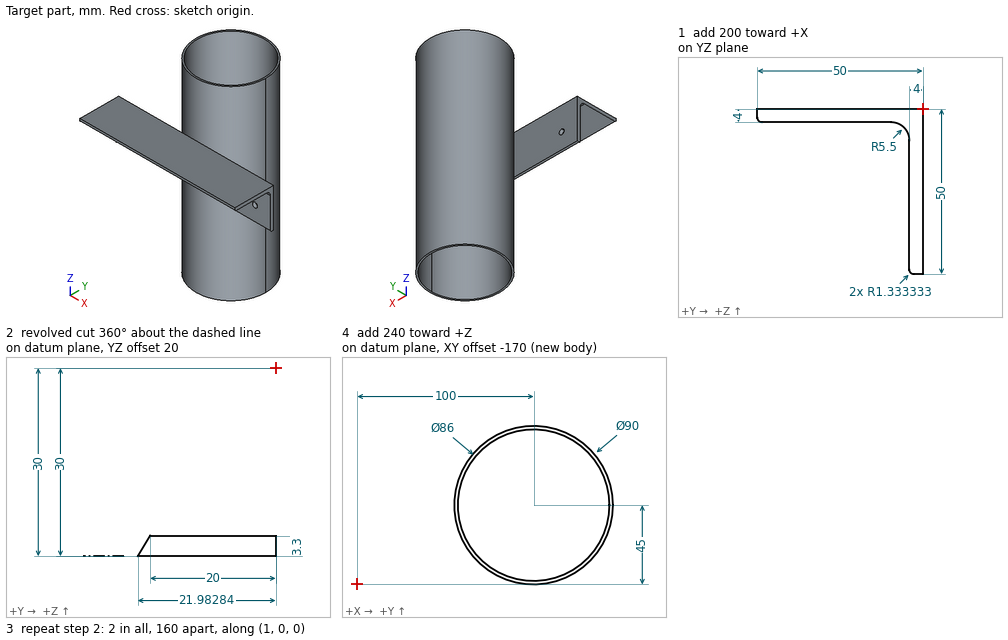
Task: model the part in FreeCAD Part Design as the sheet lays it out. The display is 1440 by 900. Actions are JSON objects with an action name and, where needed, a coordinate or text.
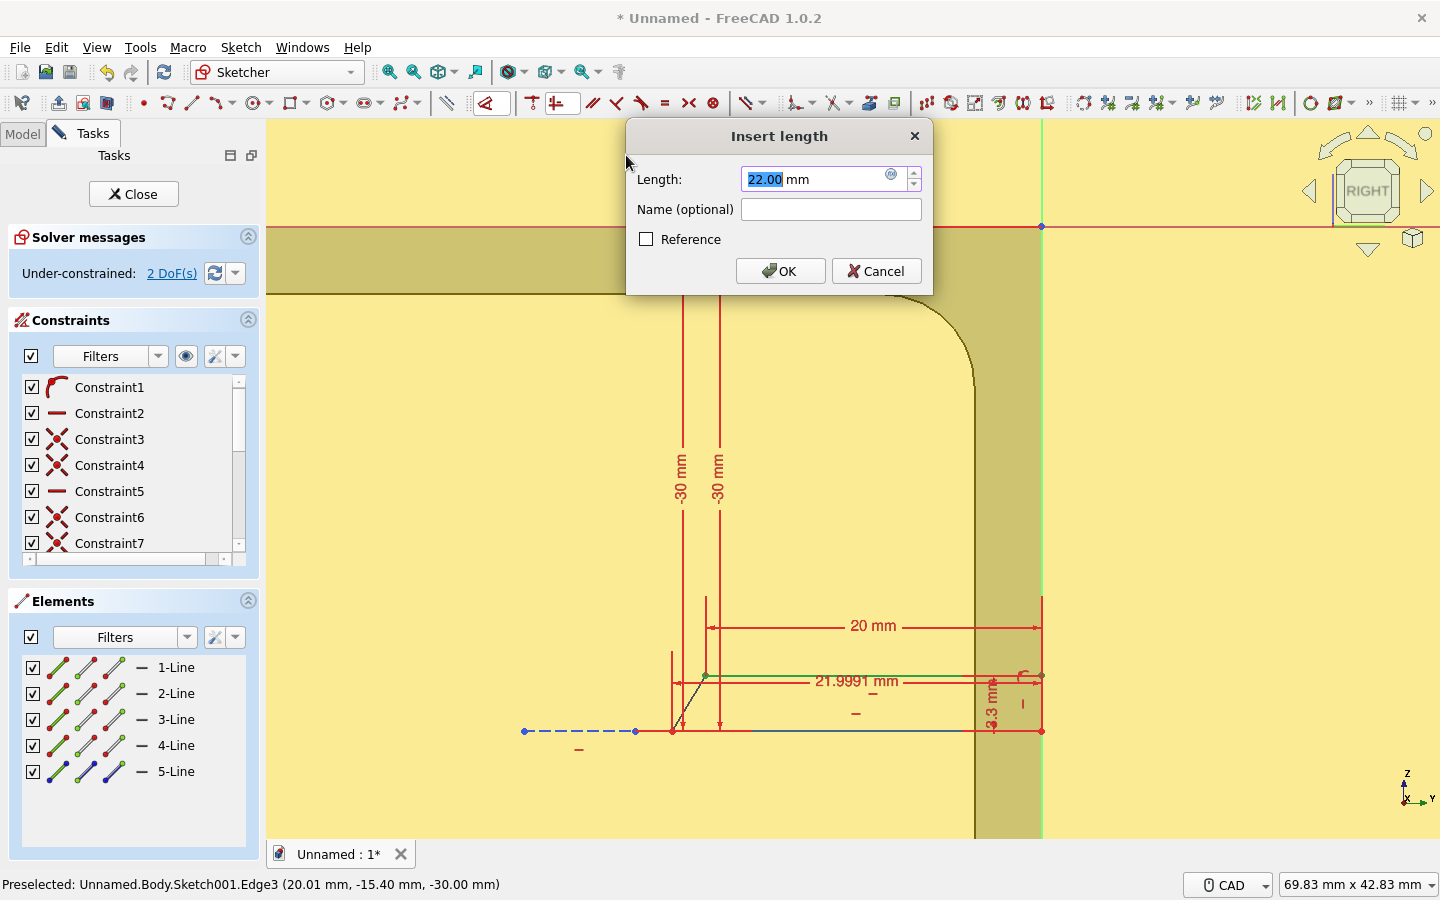
{"action": "type", "text": "21.98284"}
{"action": "key", "text": "Return"}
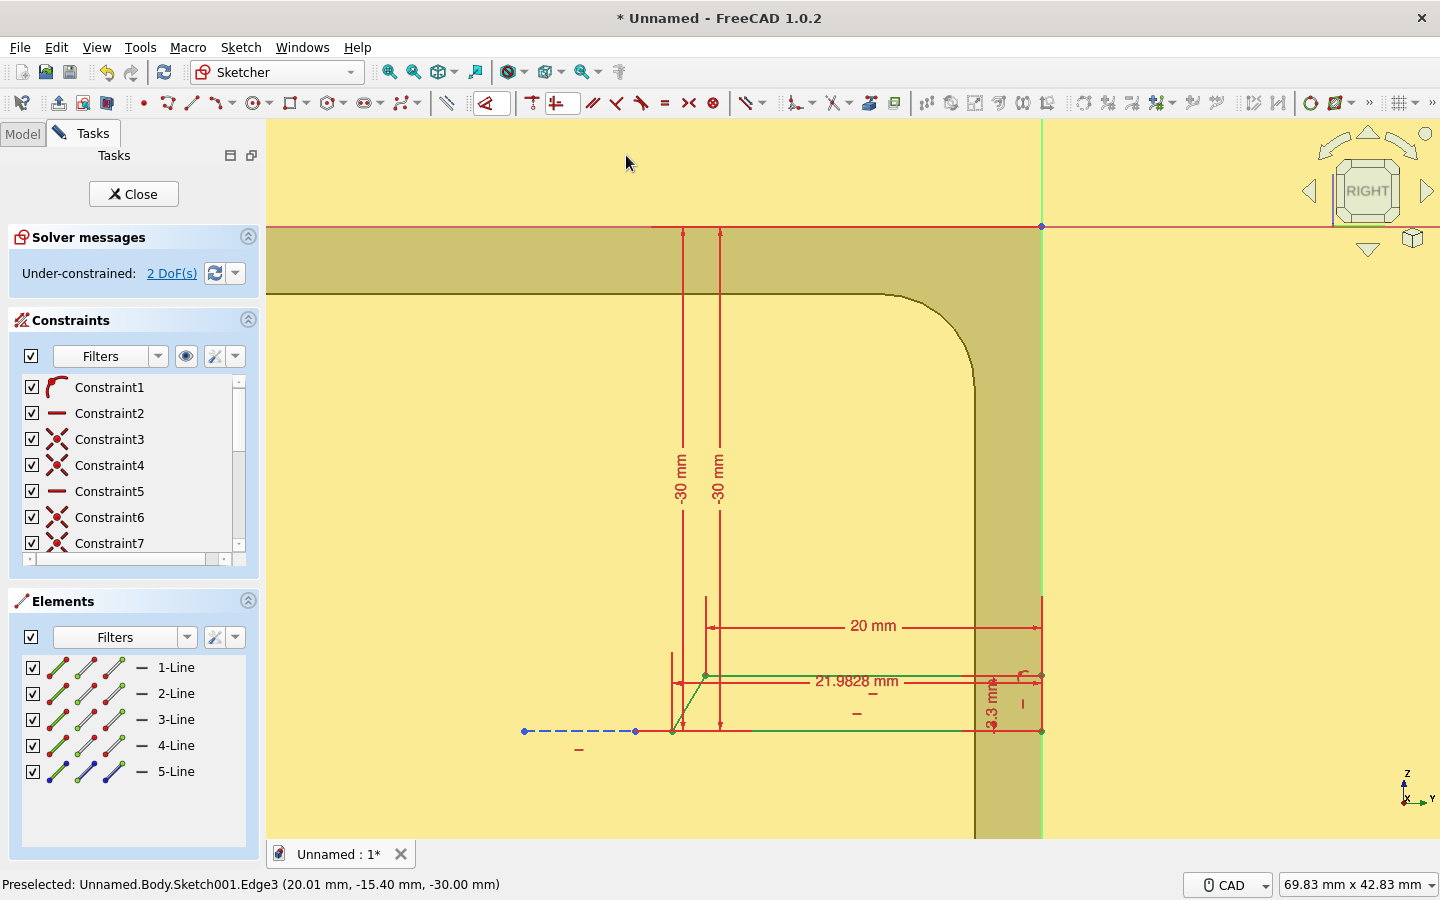
{"action": "left_click", "coordinate": [134, 194]}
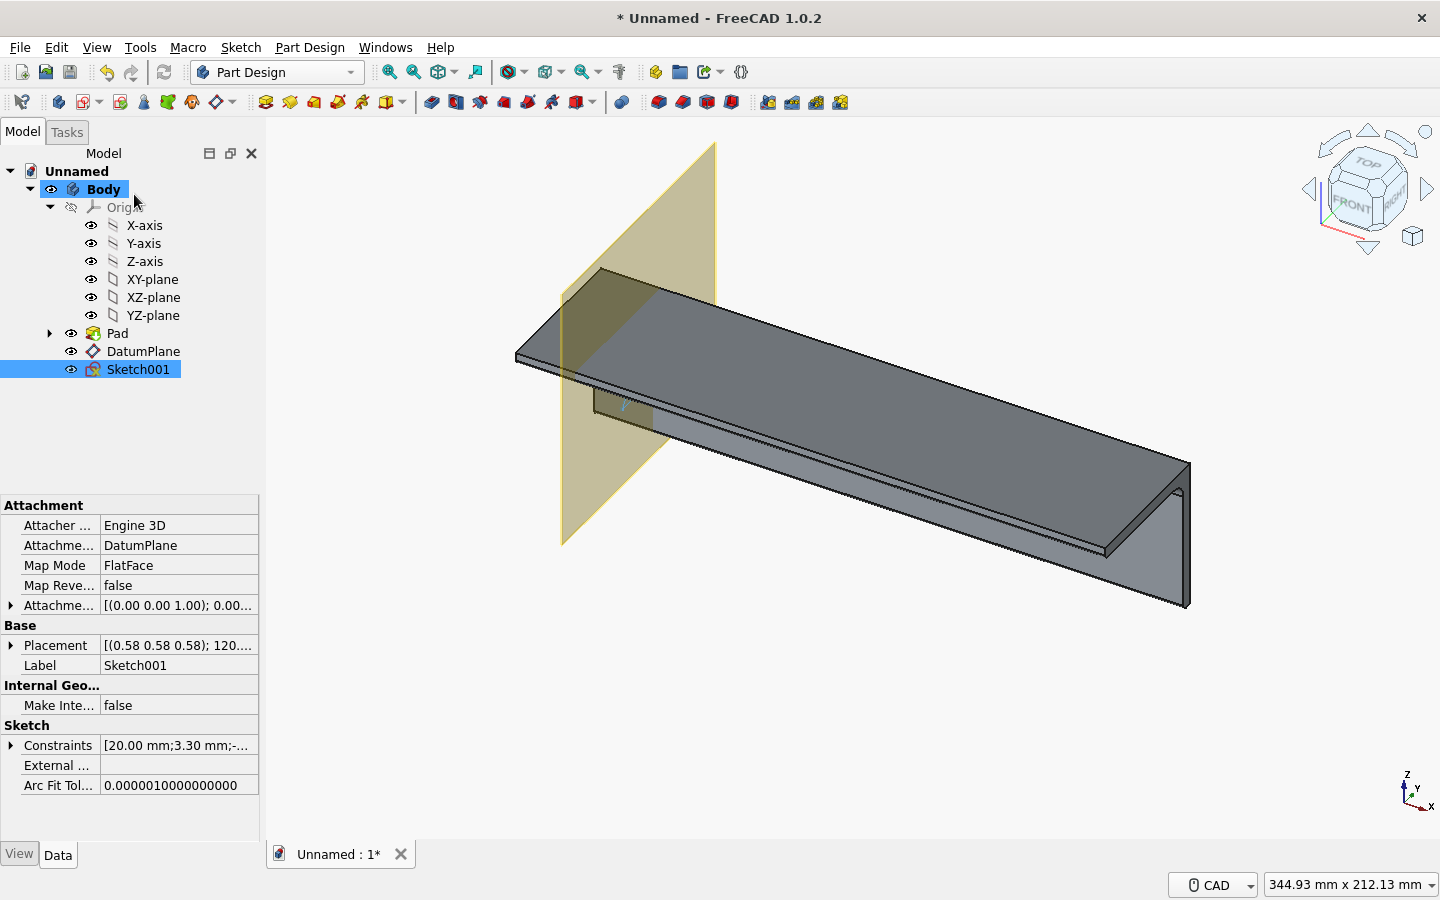
{"action": "left_click", "coordinate": [480, 102]}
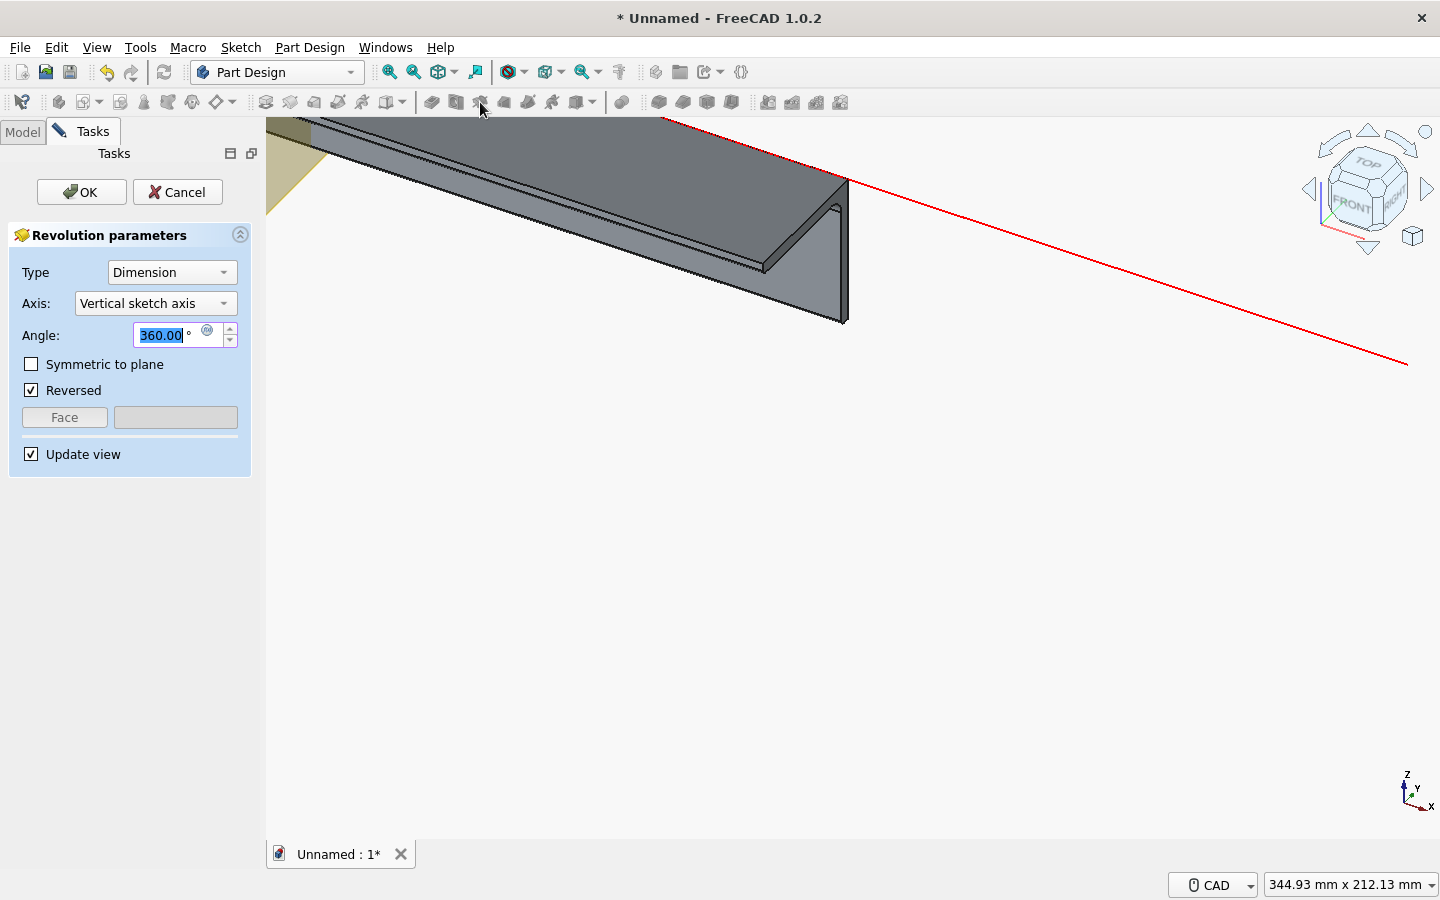
{"action": "left_click", "coordinate": [156, 304]}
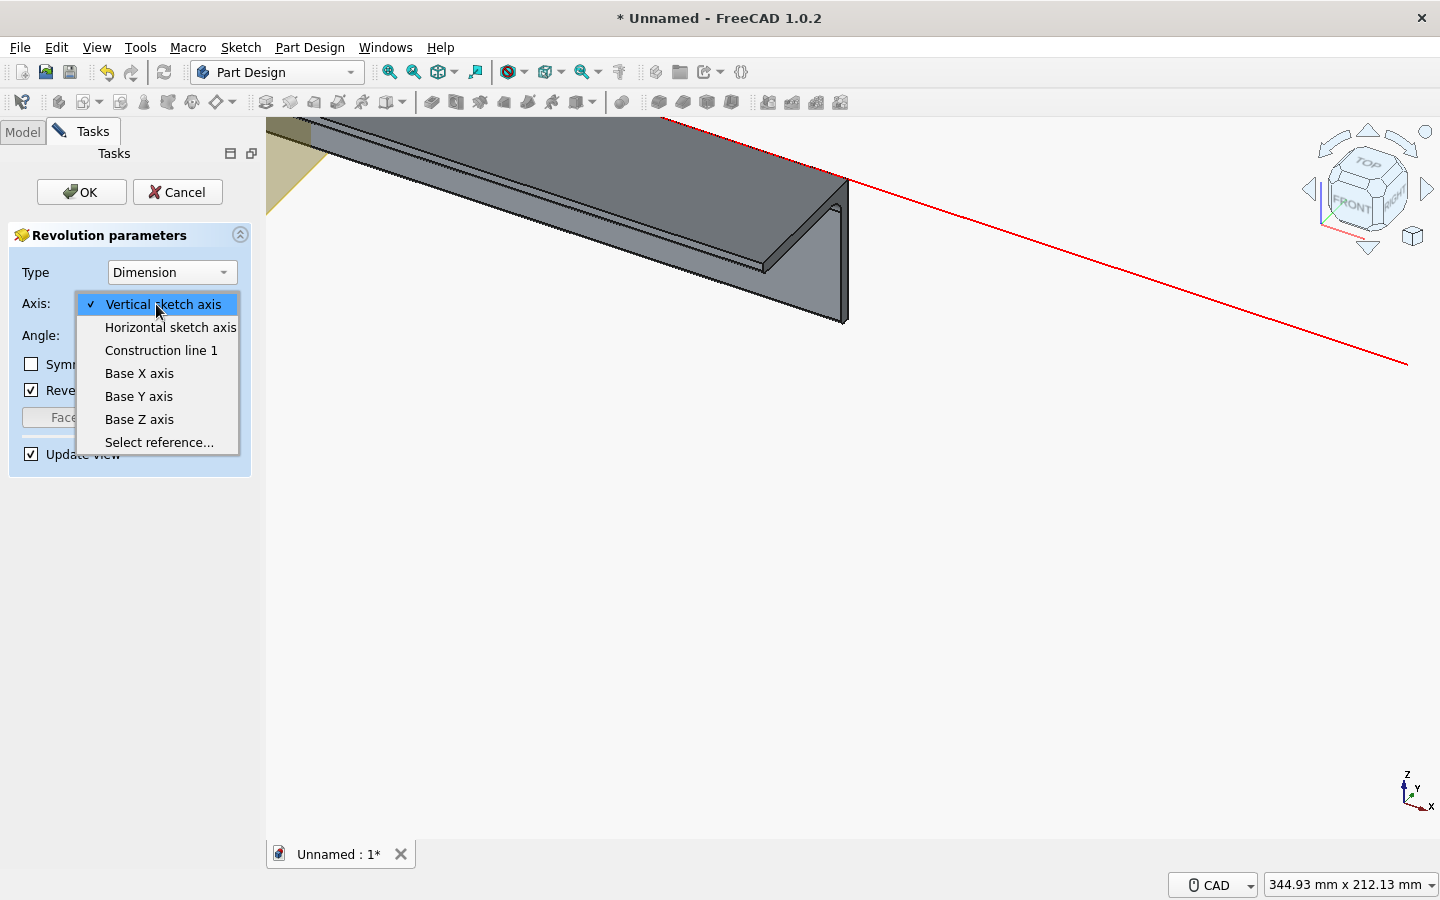
{"action": "left_click", "coordinate": [156, 350]}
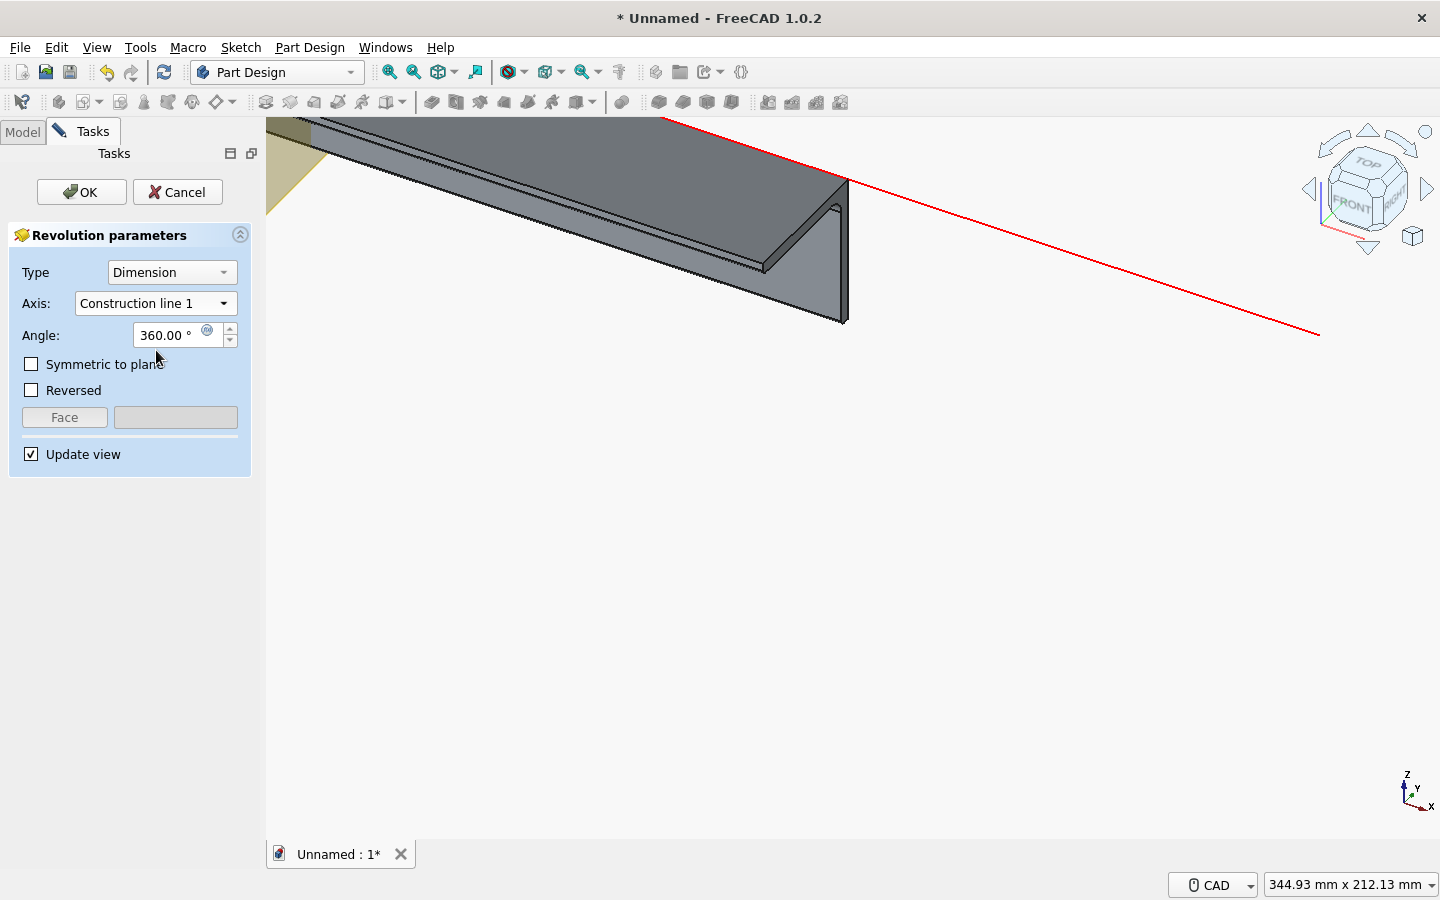
{"action": "left_click", "coordinate": [82, 192]}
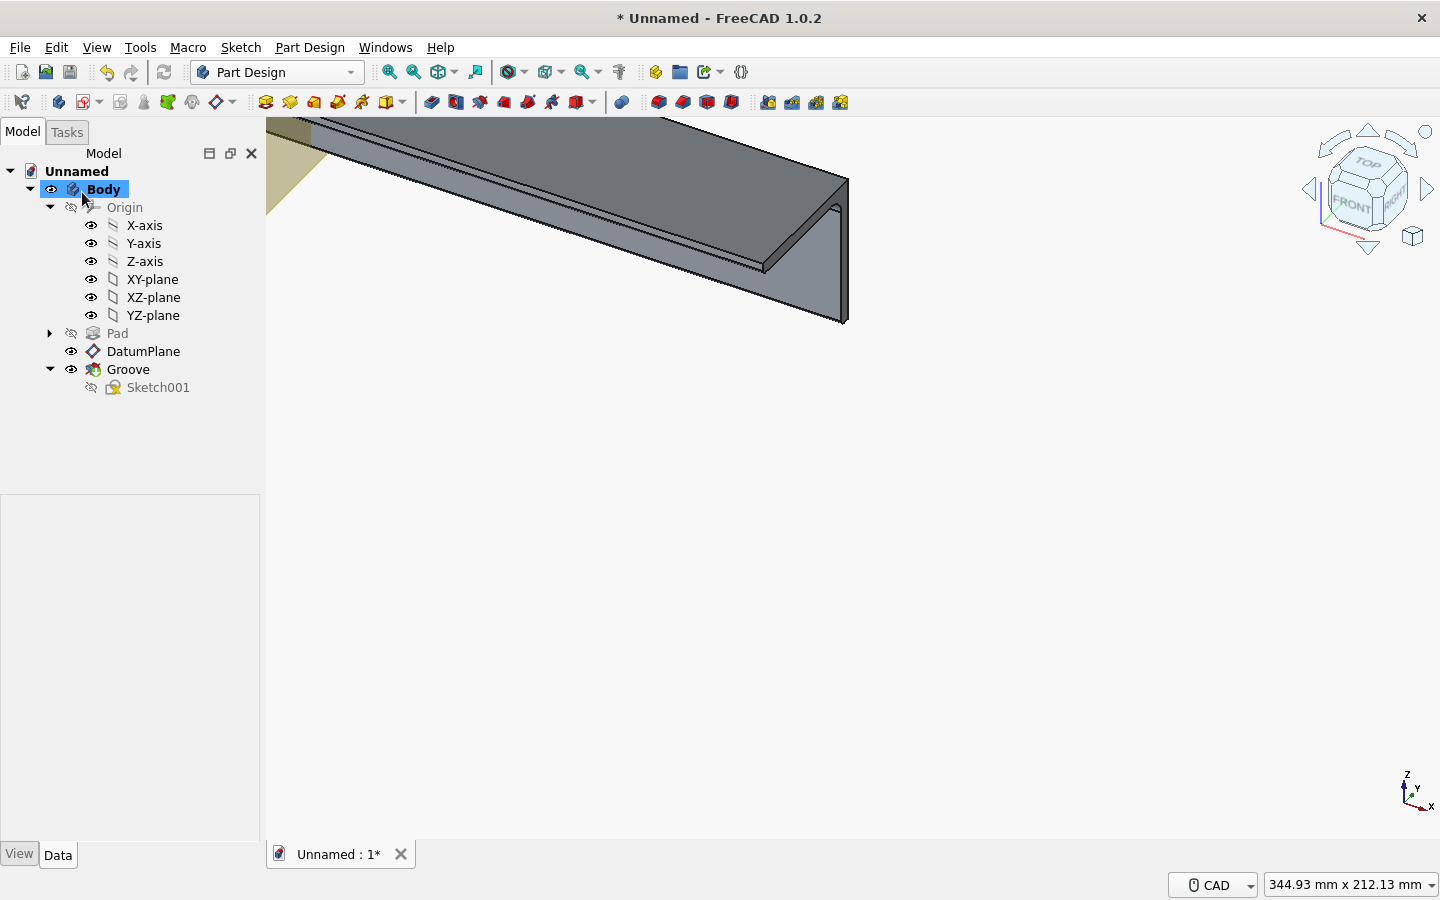
{"action": "left_click", "coordinate": [116, 351]}
{"action": "key", "text": "space"}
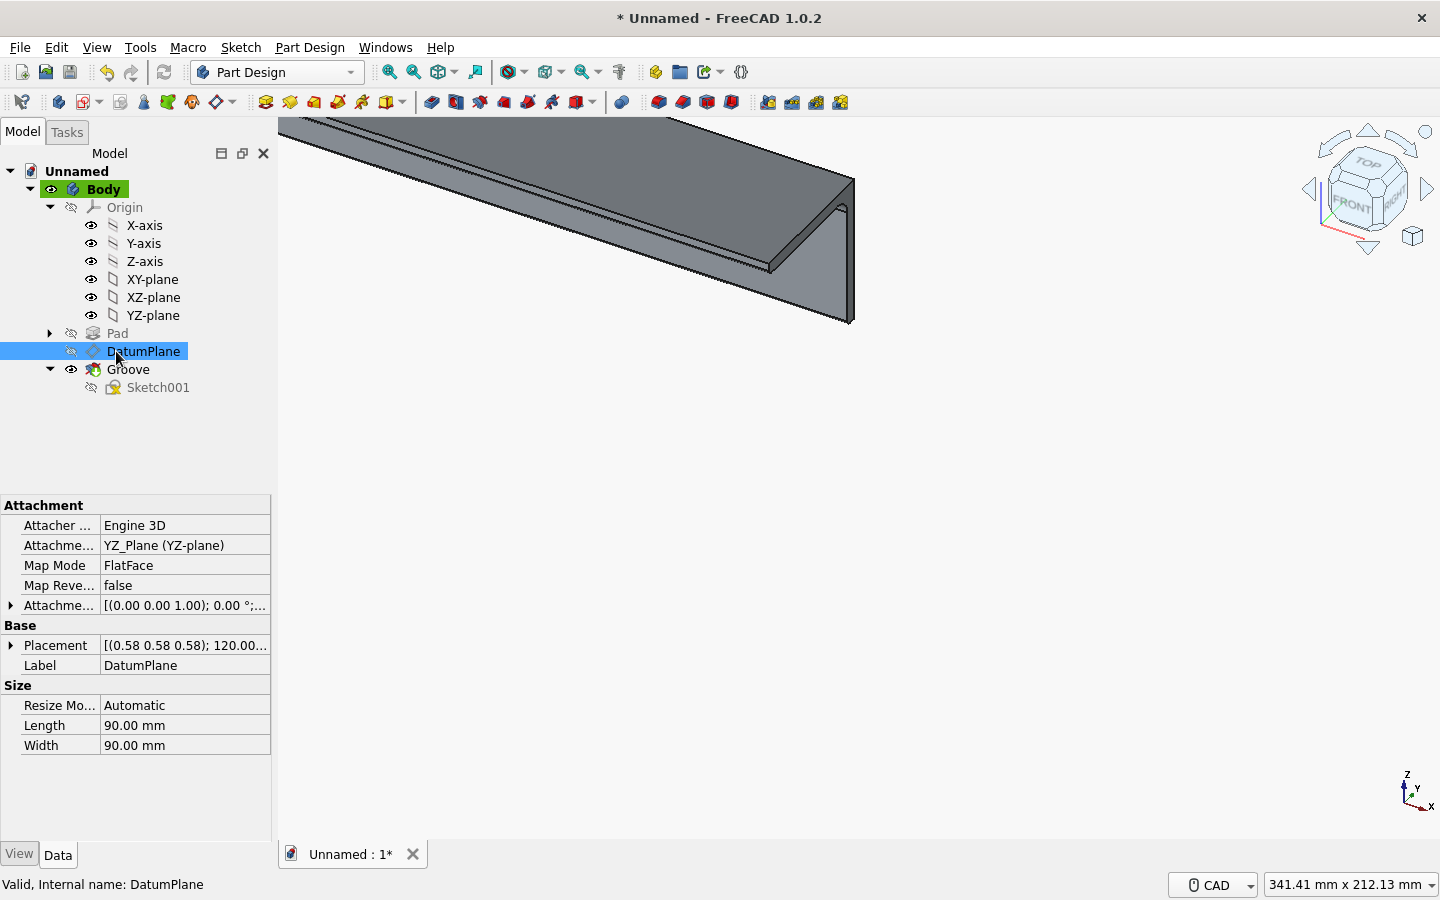
{"action": "left_click", "coordinate": [390, 72]}